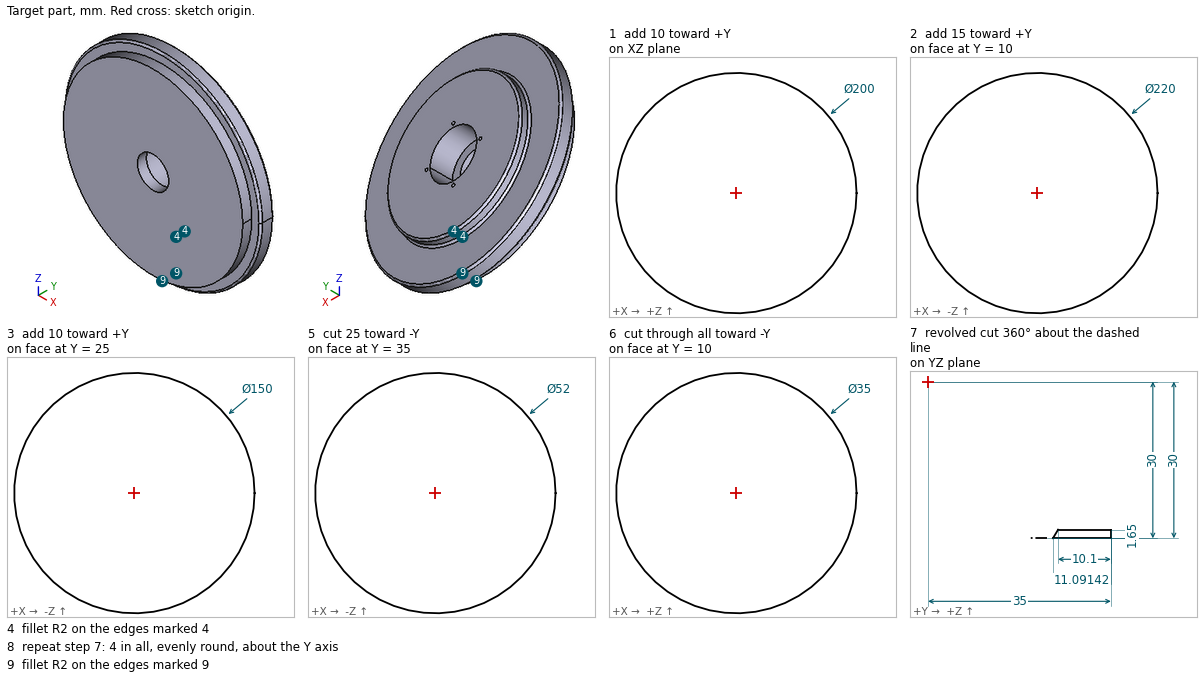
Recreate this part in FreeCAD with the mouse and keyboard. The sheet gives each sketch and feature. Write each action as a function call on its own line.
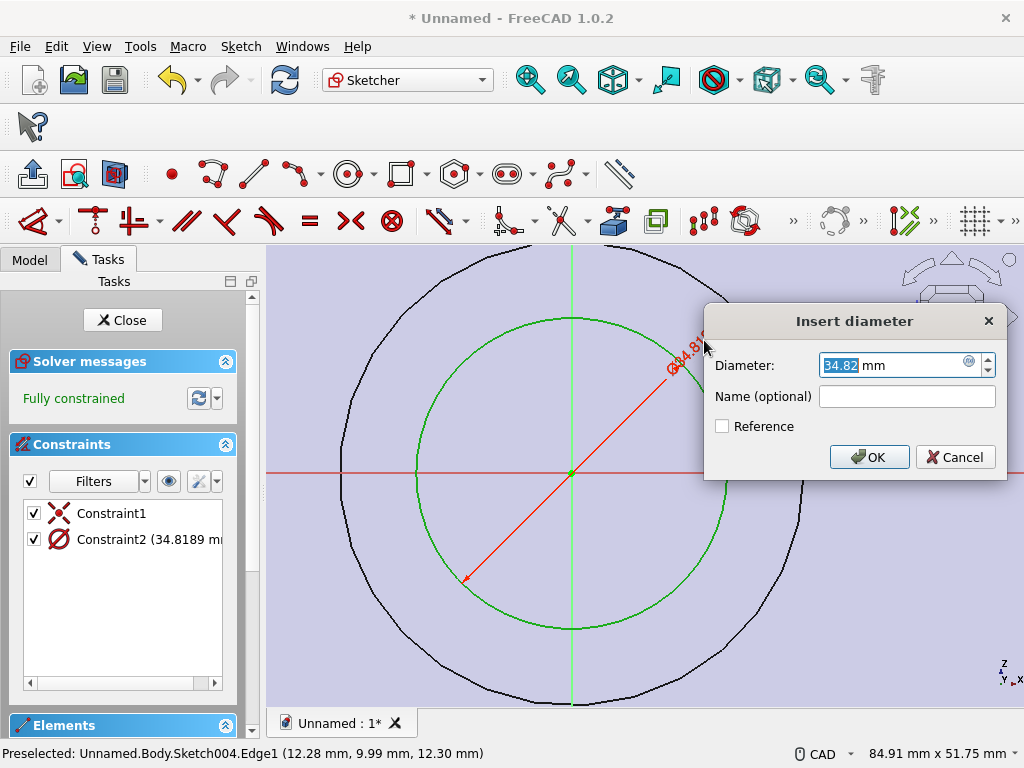
text(35)
key(Return)
key(Escape)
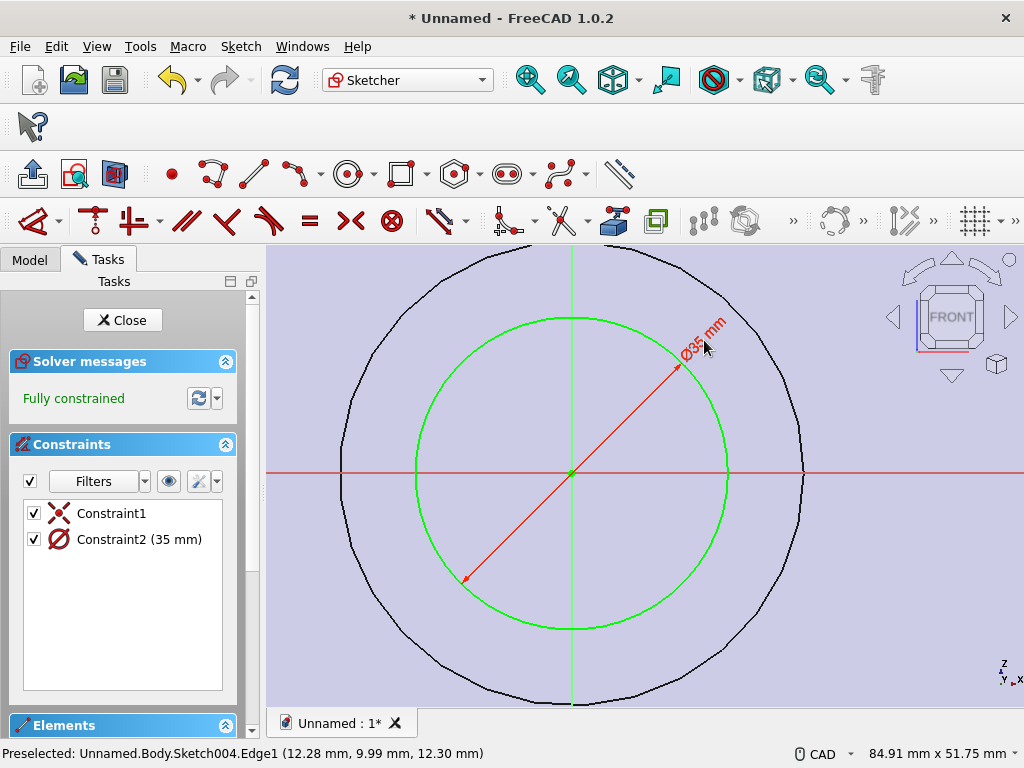
click(123, 320)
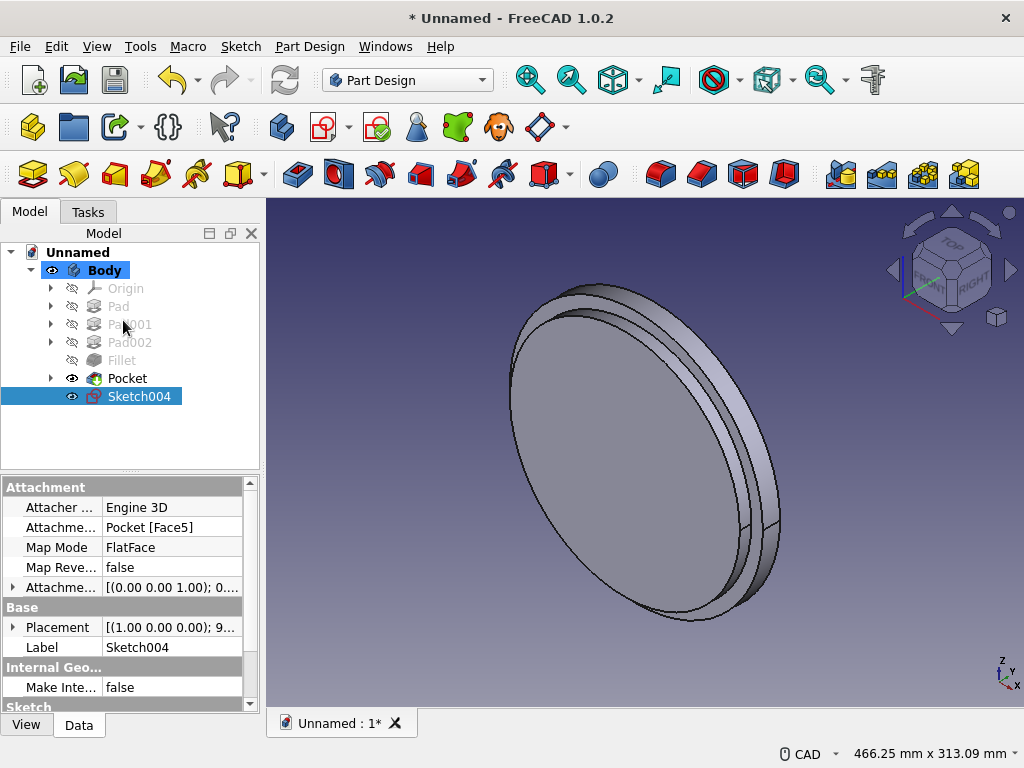
click(298, 174)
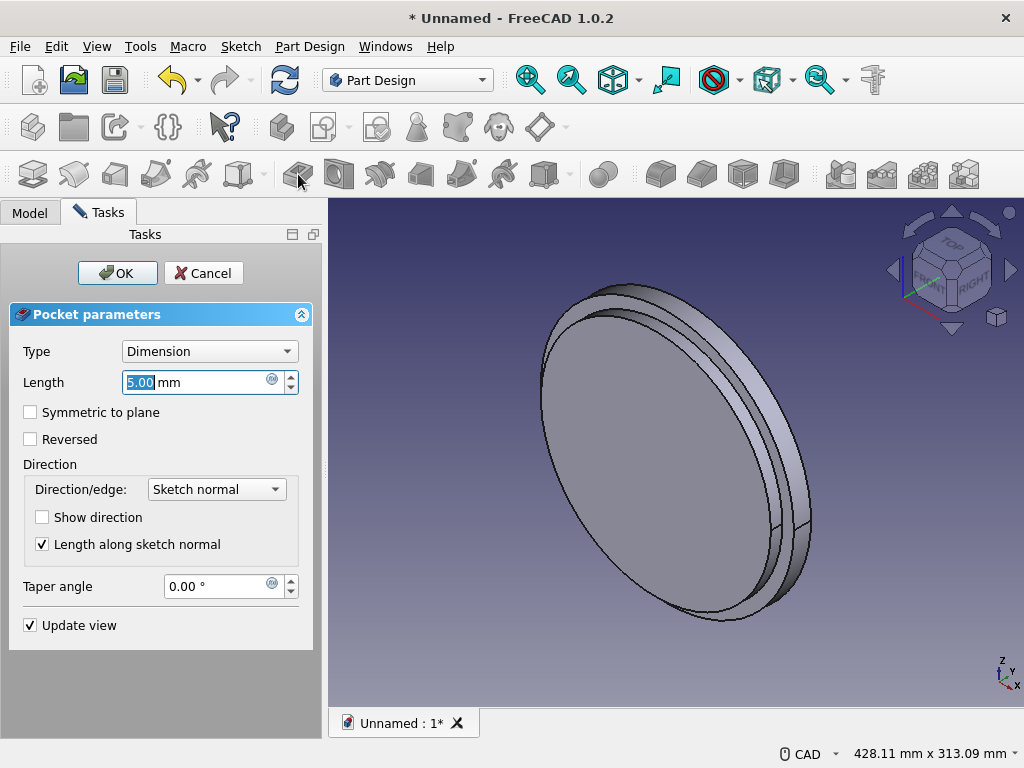
click(210, 352)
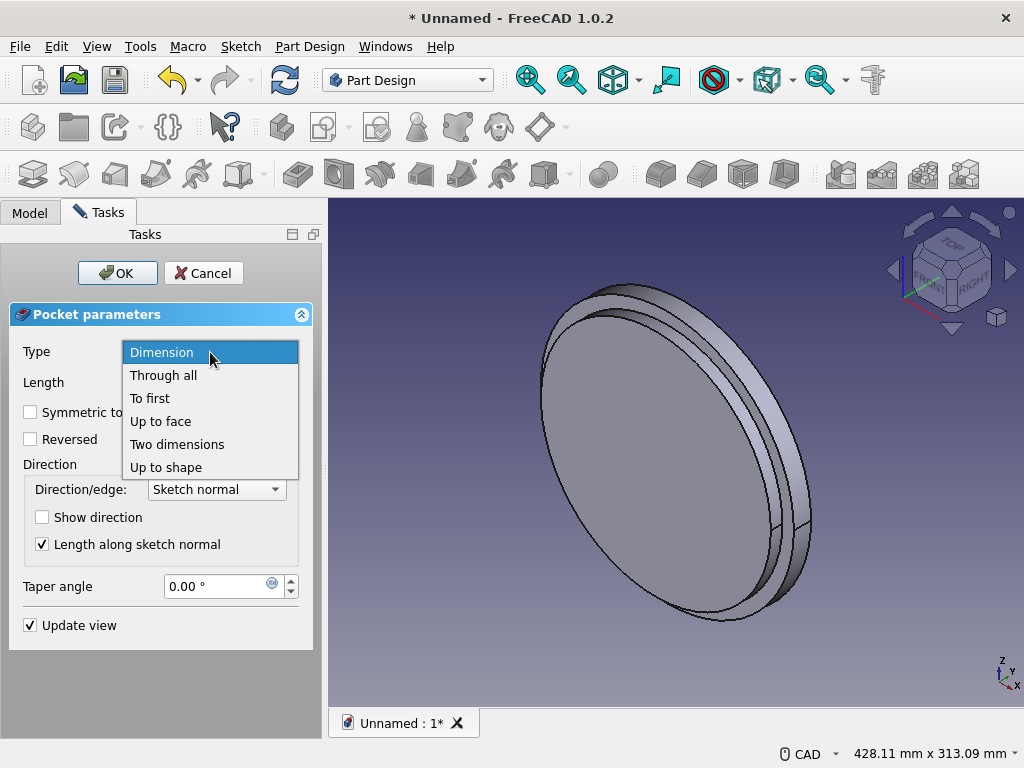
click(208, 376)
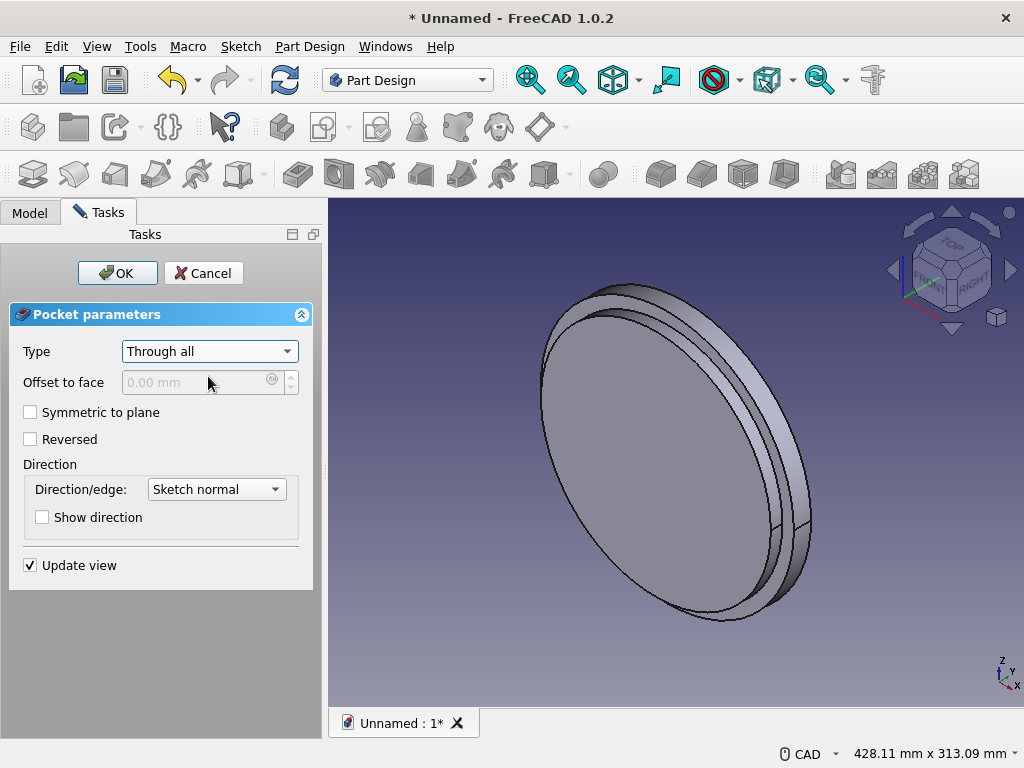
click(31, 439)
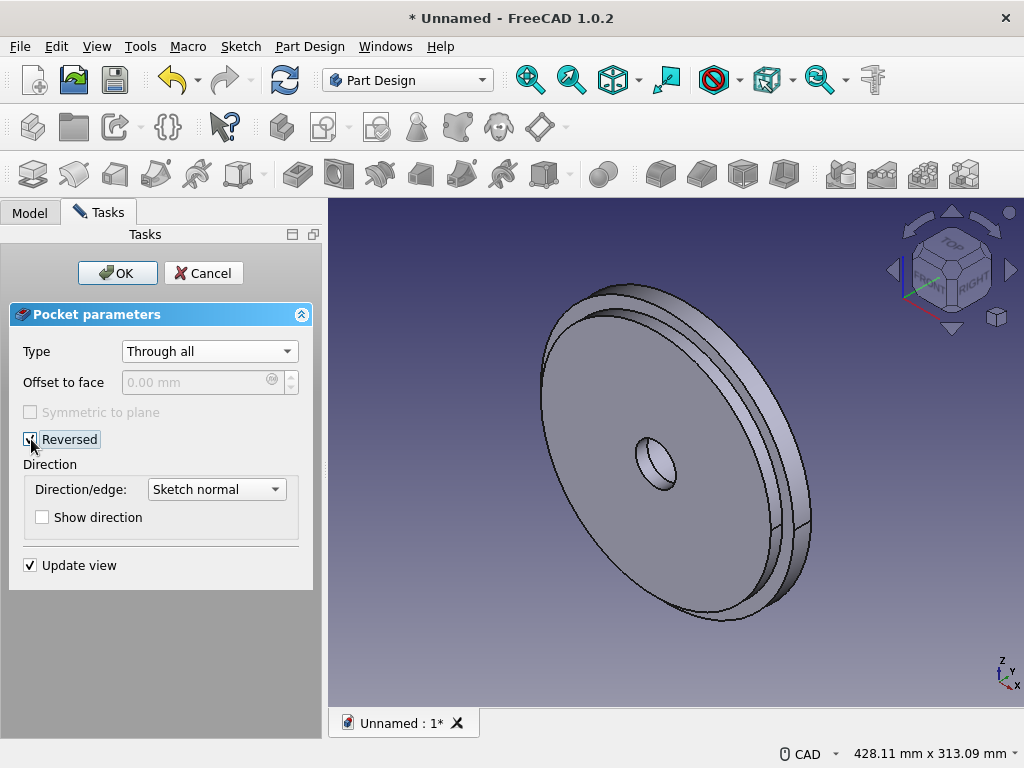
click(118, 273)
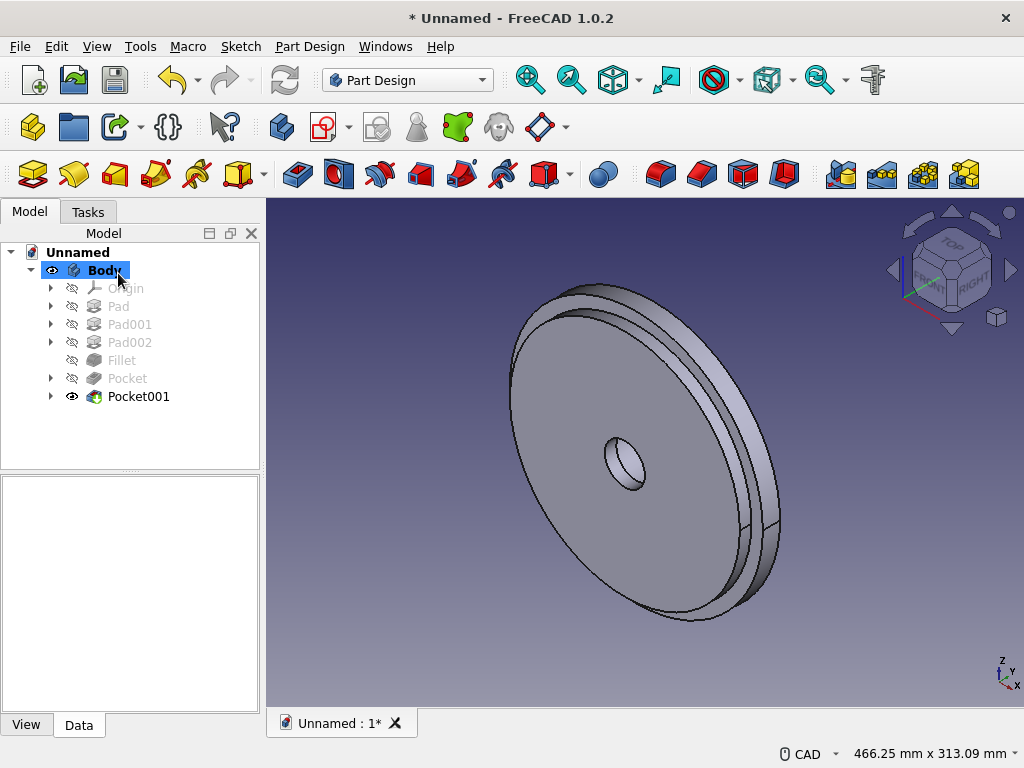
click(322, 128)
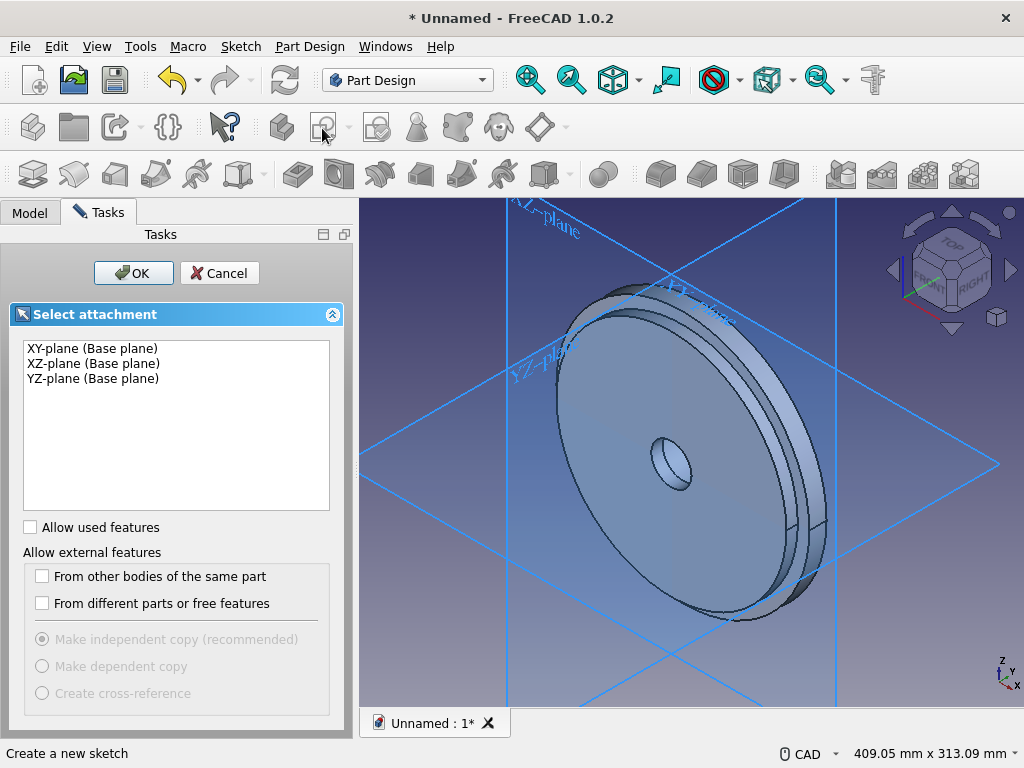
click(84, 378)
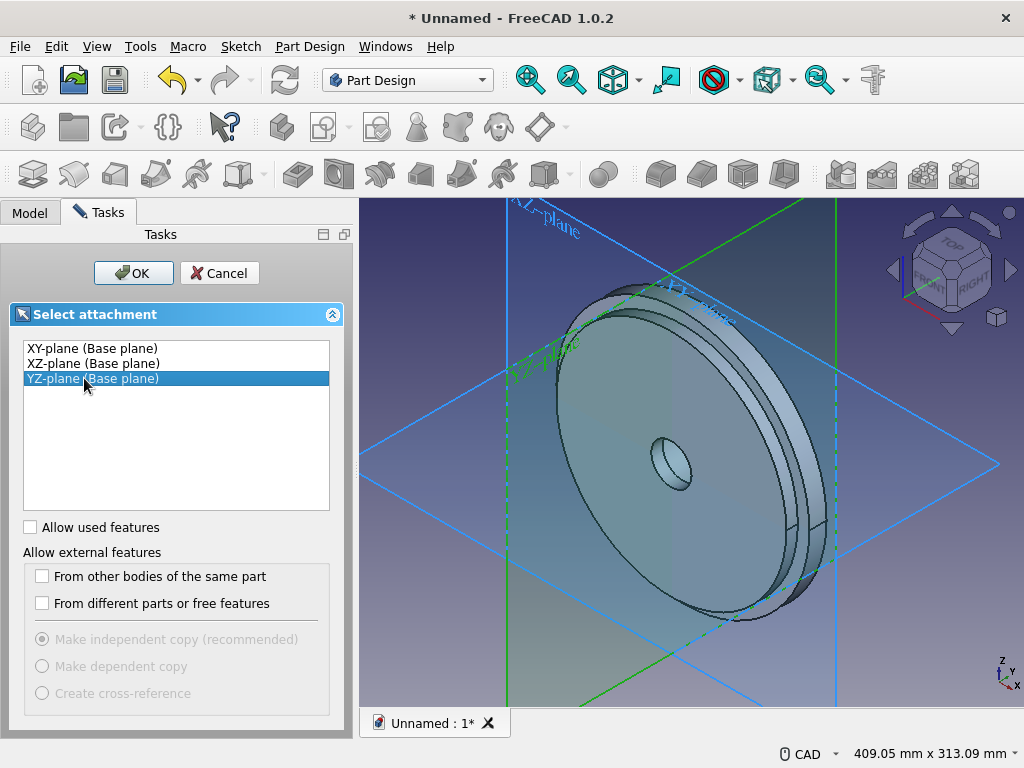
click(134, 273)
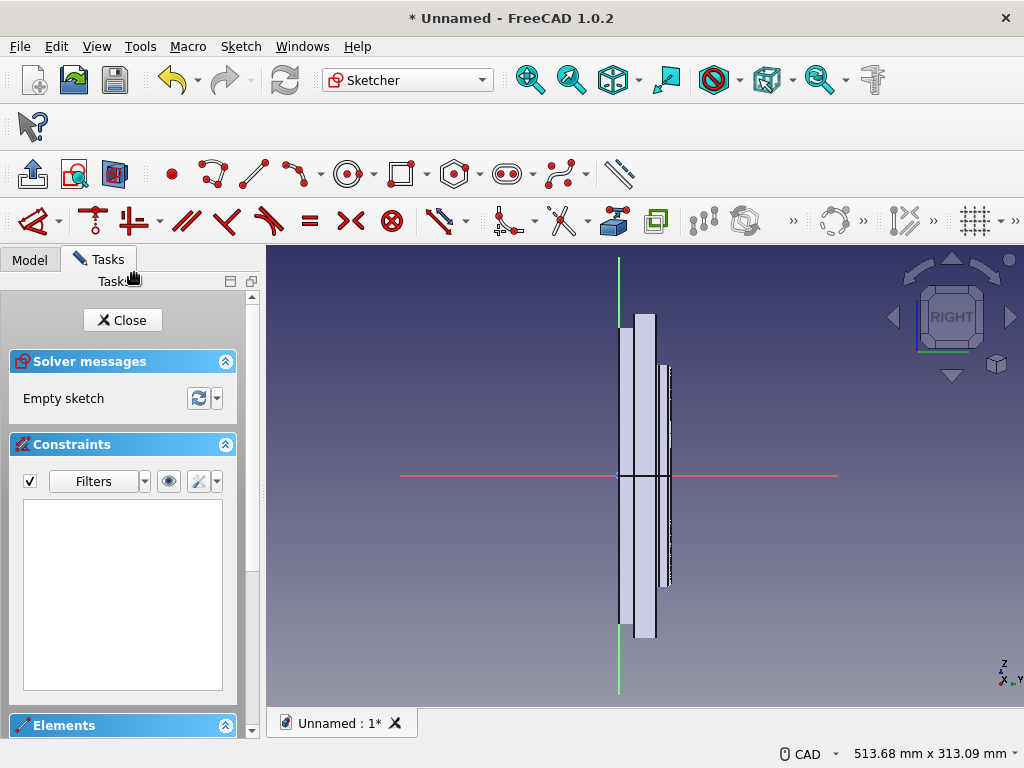
click(115, 174)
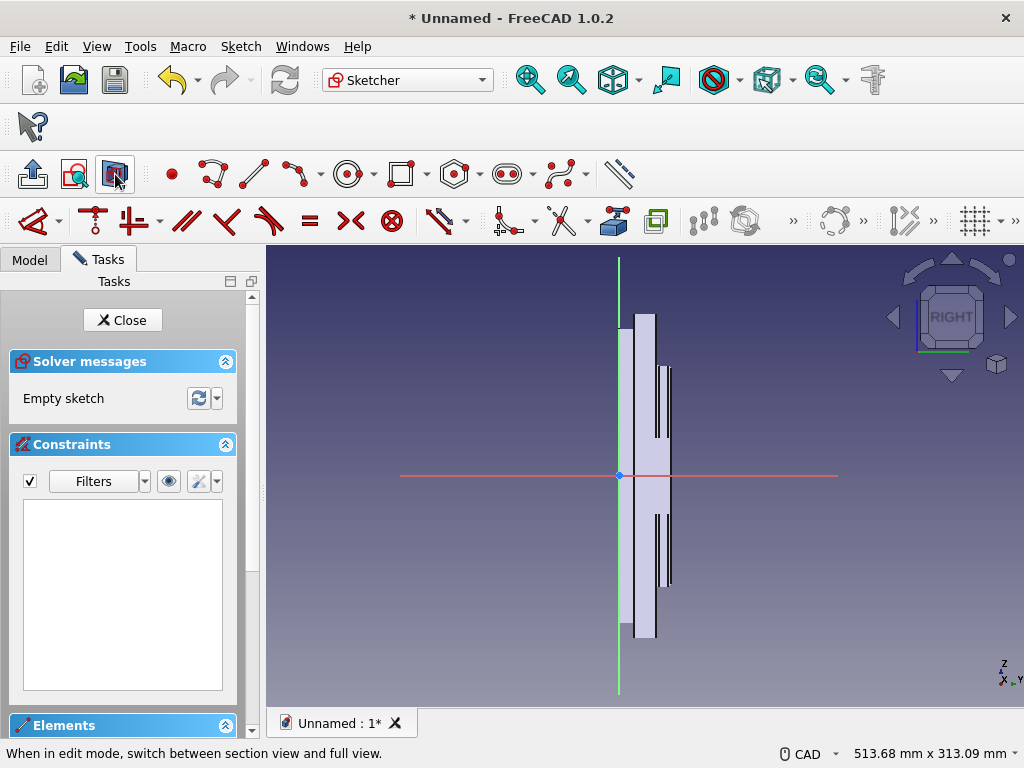
scroll(659, 503, up, 9)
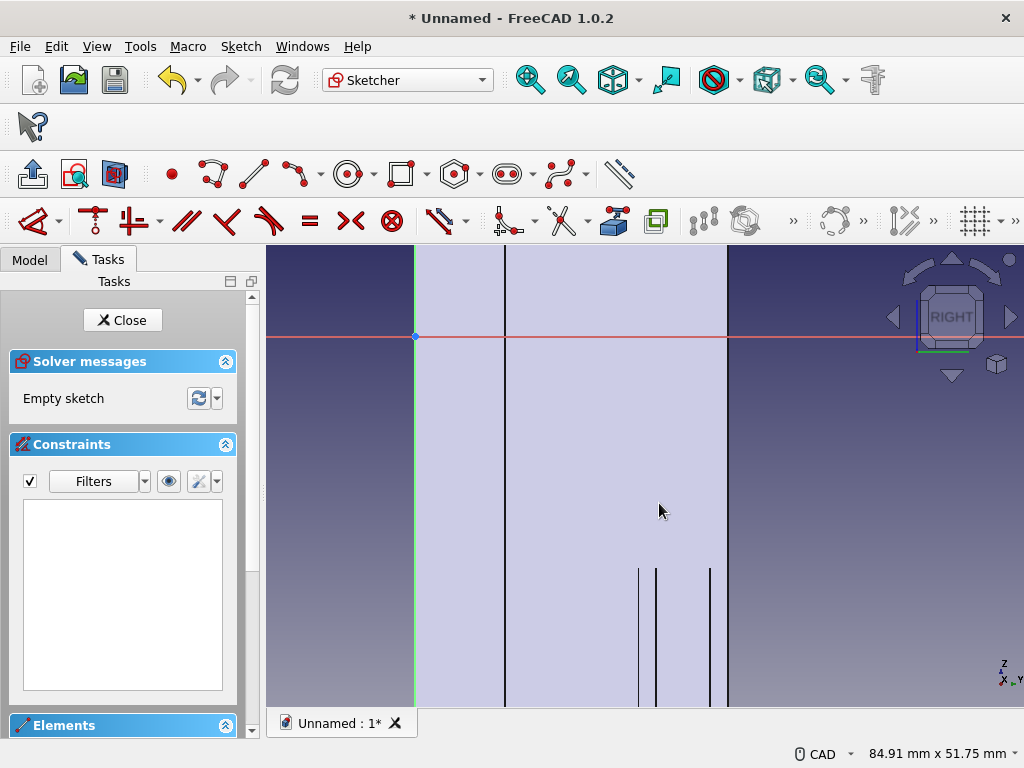
click(213, 174)